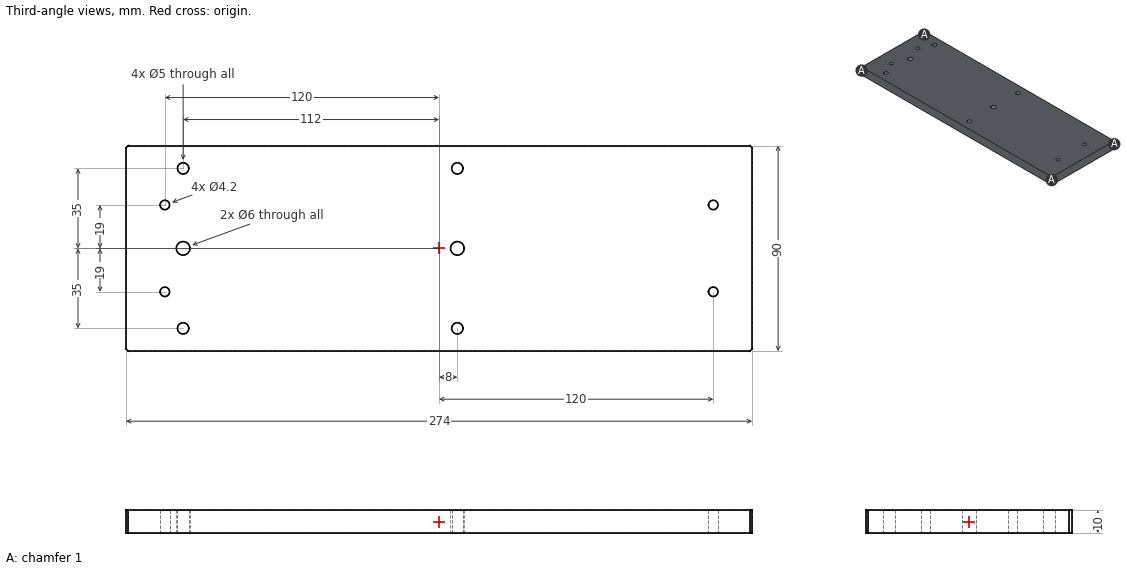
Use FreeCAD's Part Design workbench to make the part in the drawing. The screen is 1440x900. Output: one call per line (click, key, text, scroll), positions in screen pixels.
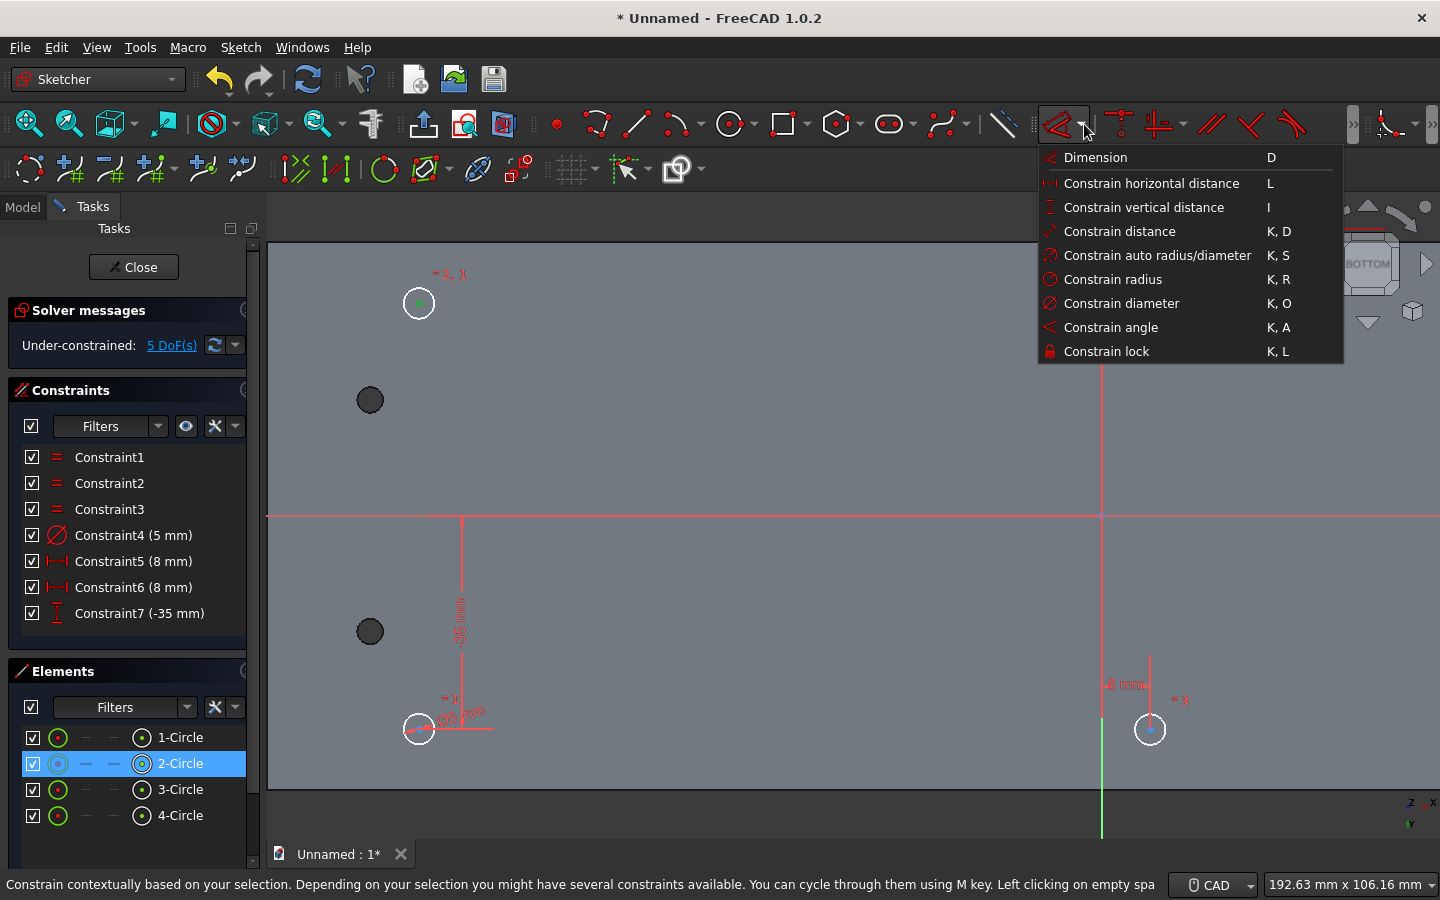
click(1191, 207)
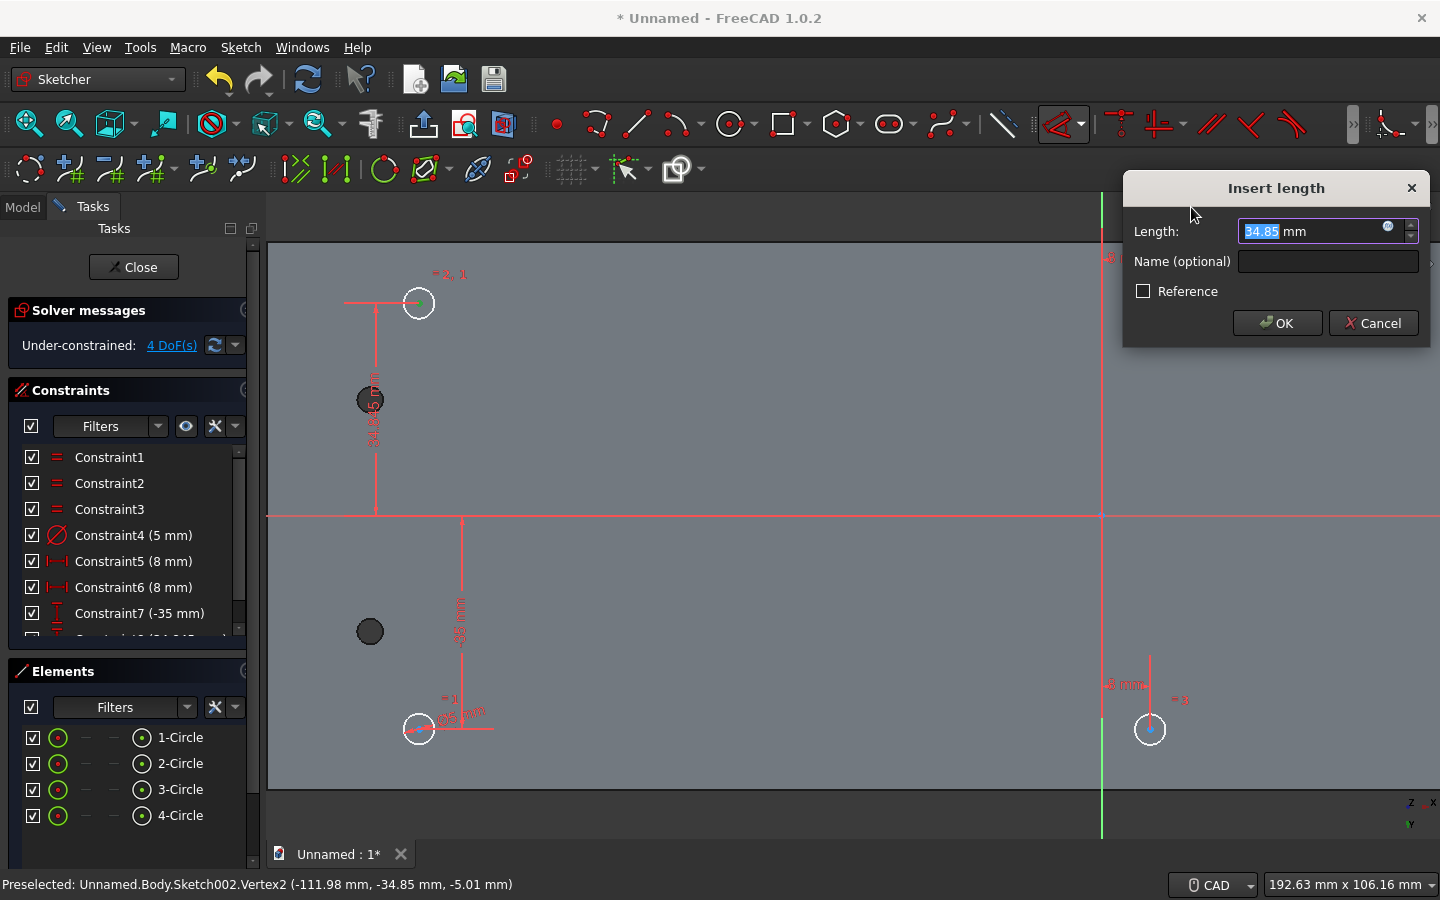
text(35)
key(Return)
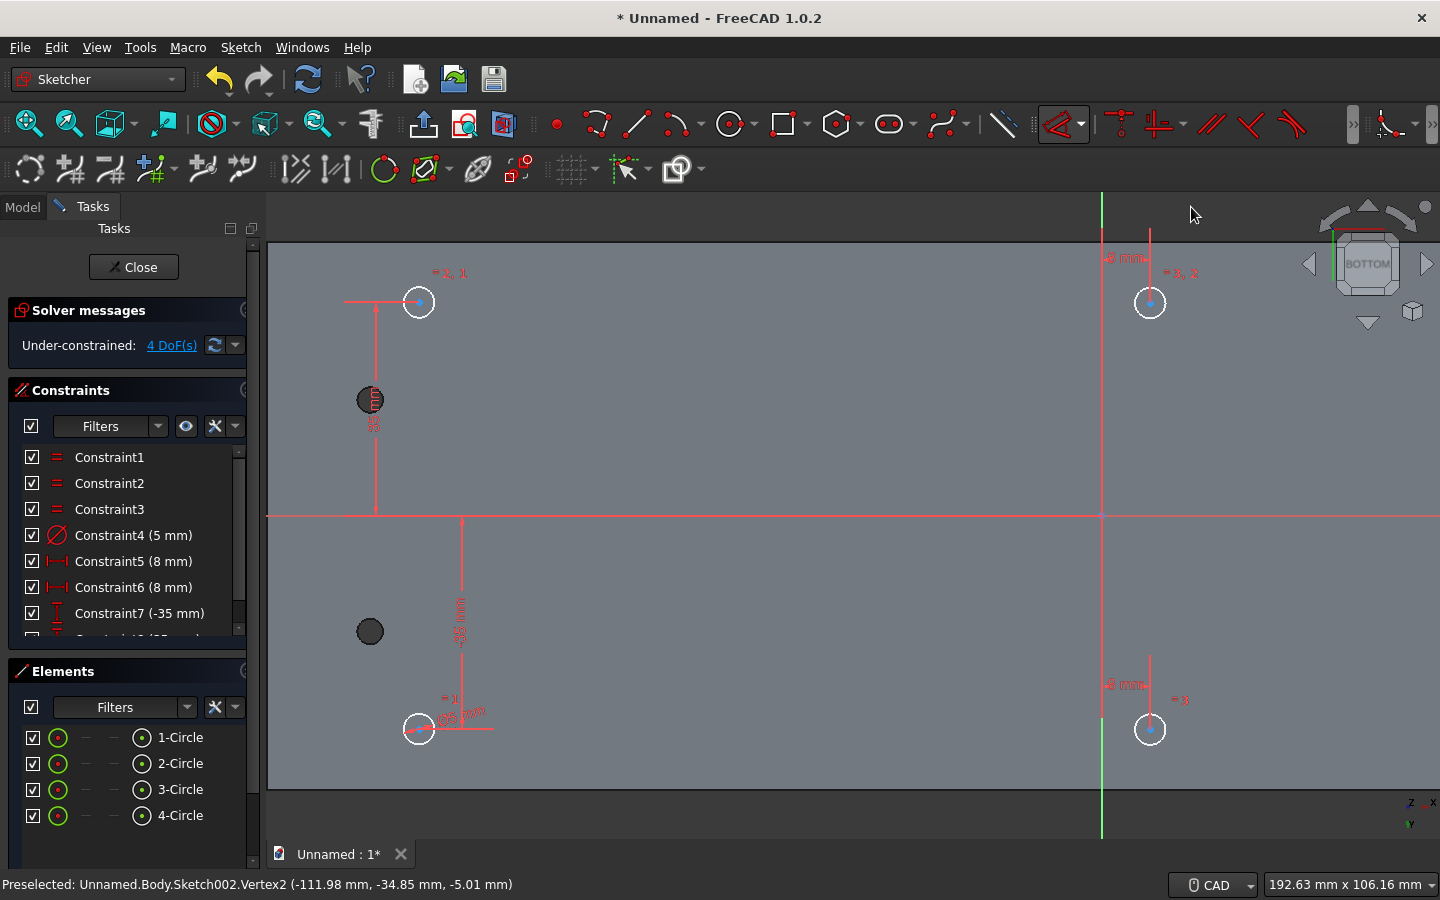
click(1150, 303)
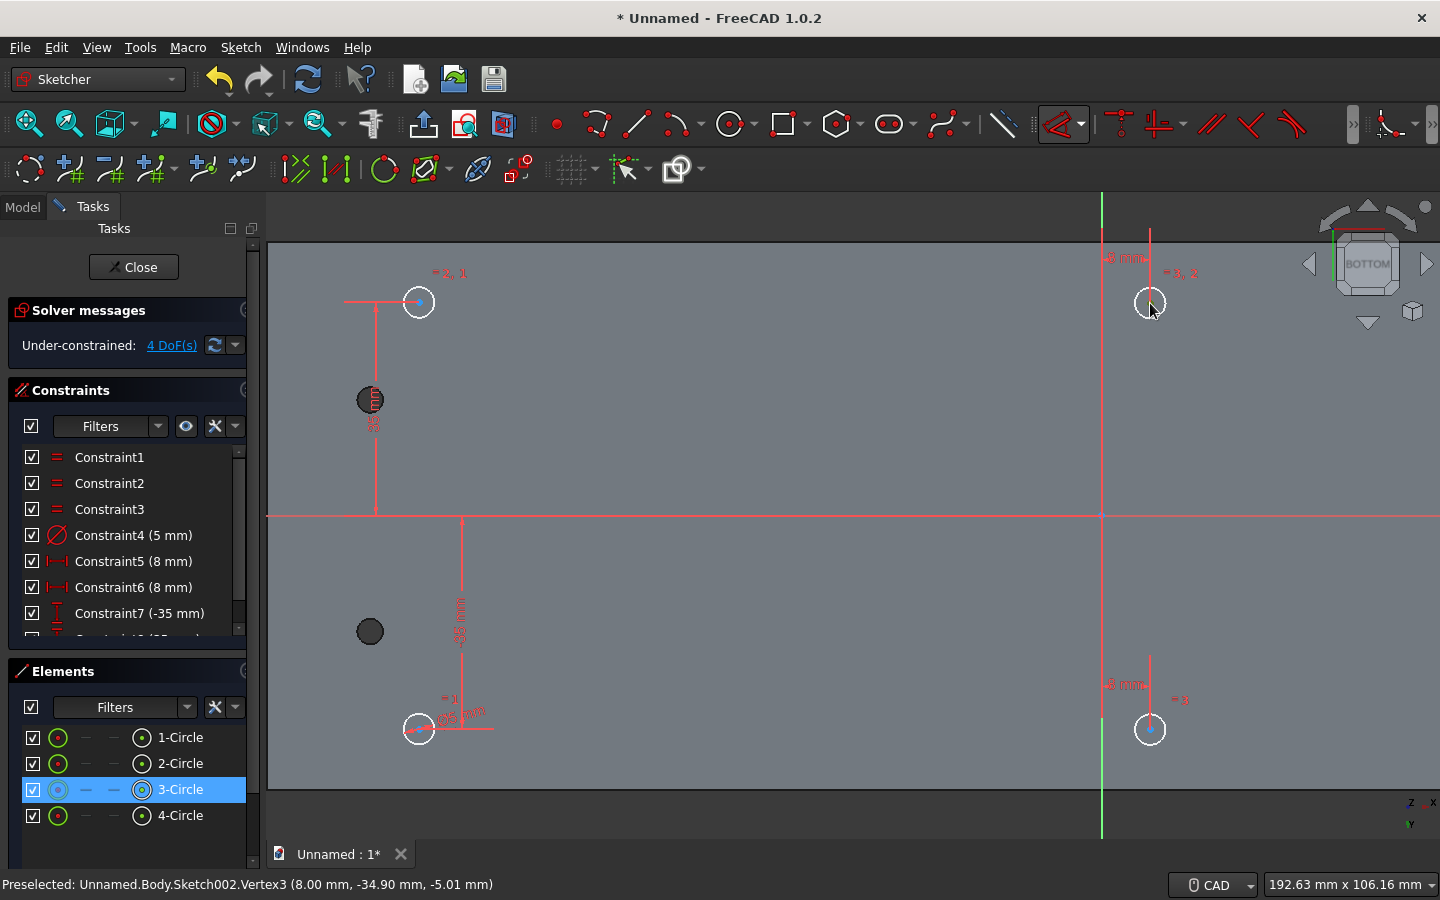
key(i)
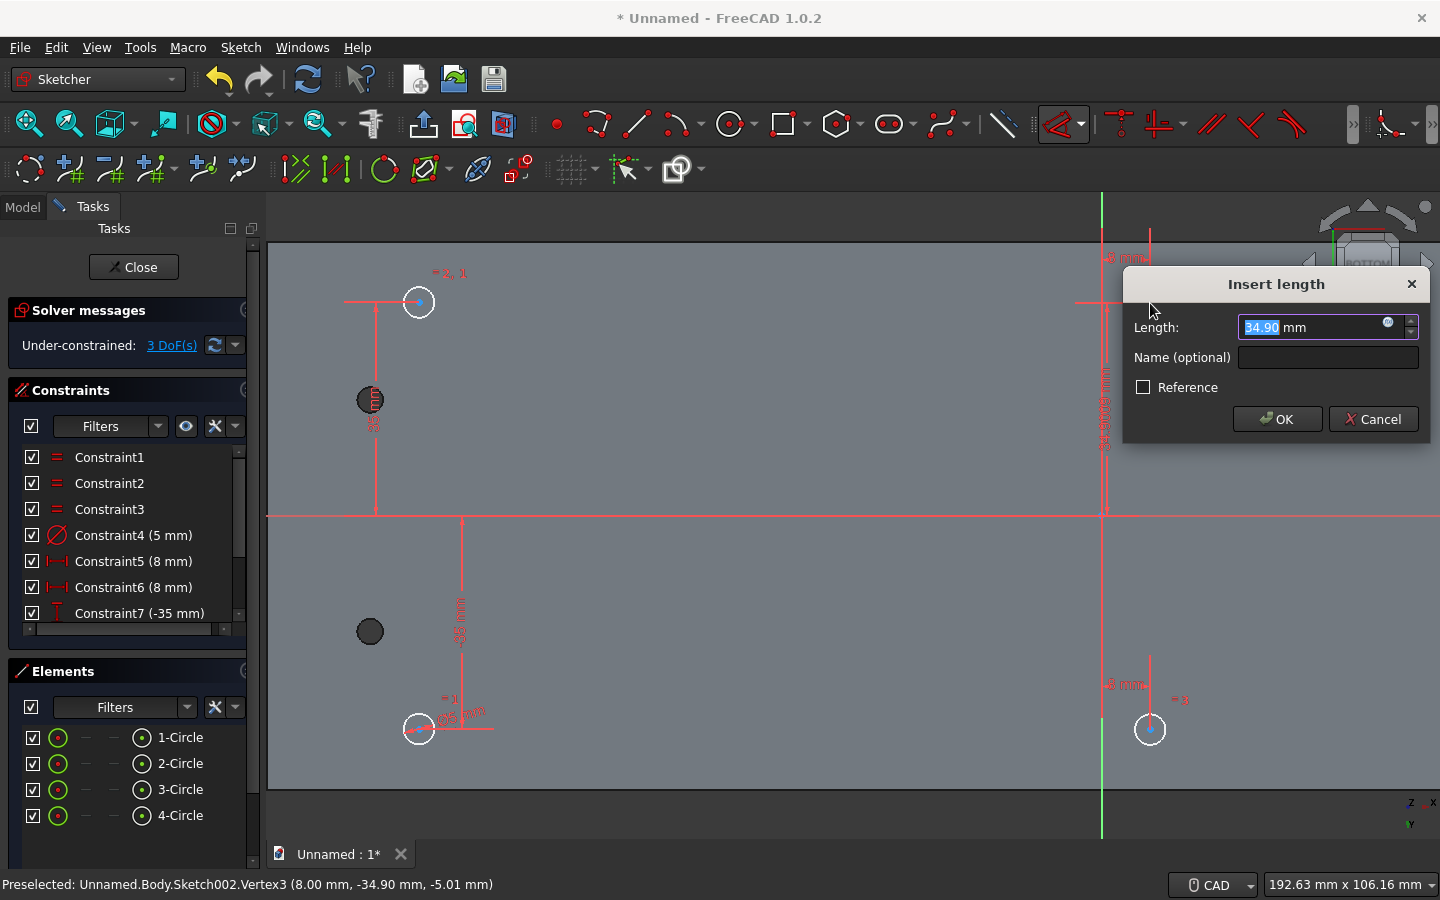
text(35)
key(Return)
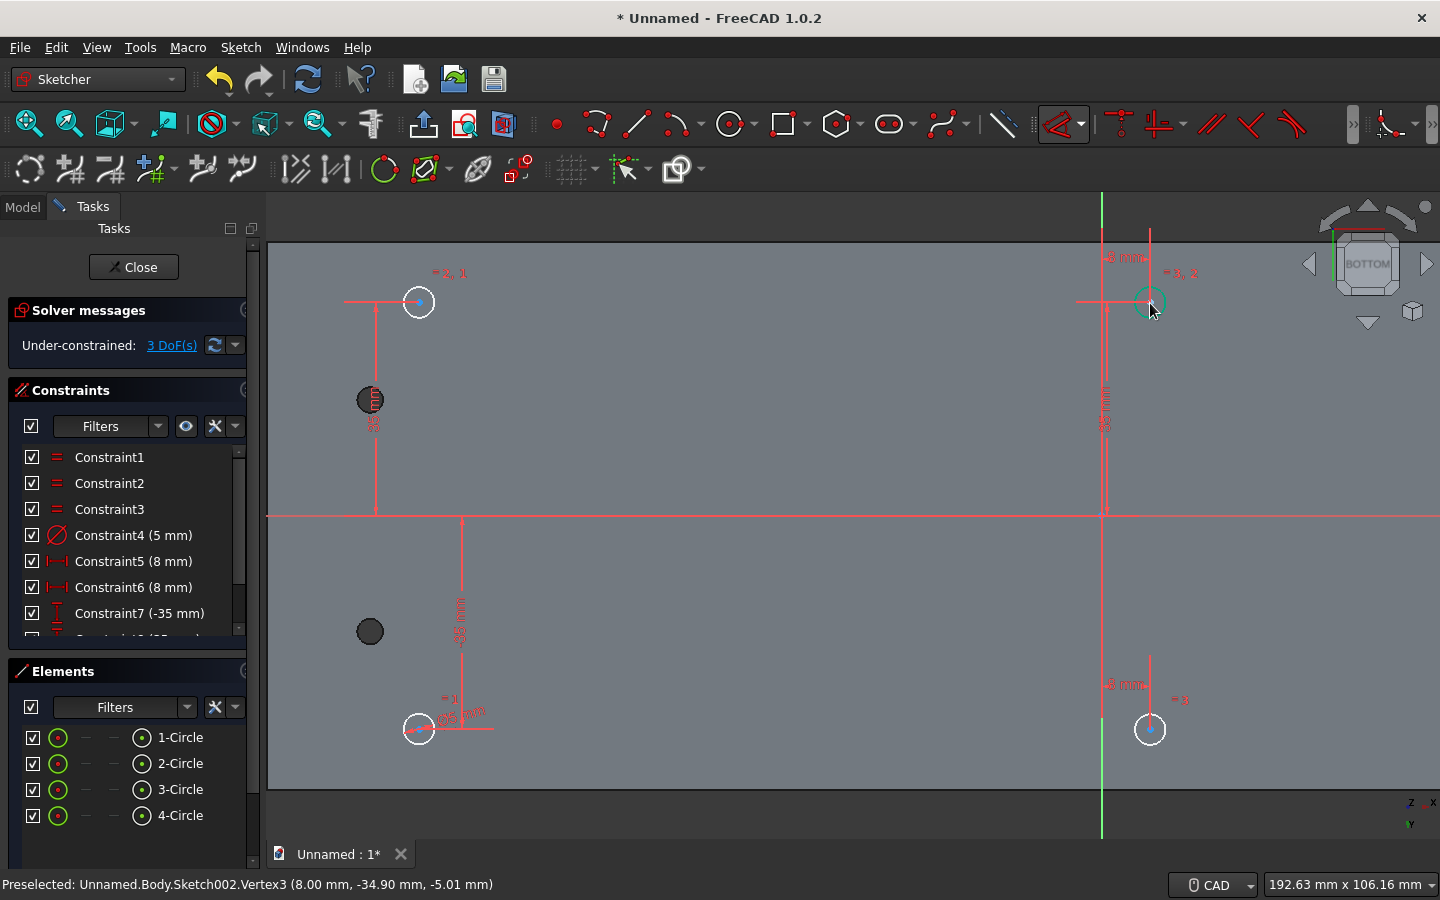
click(1150, 730)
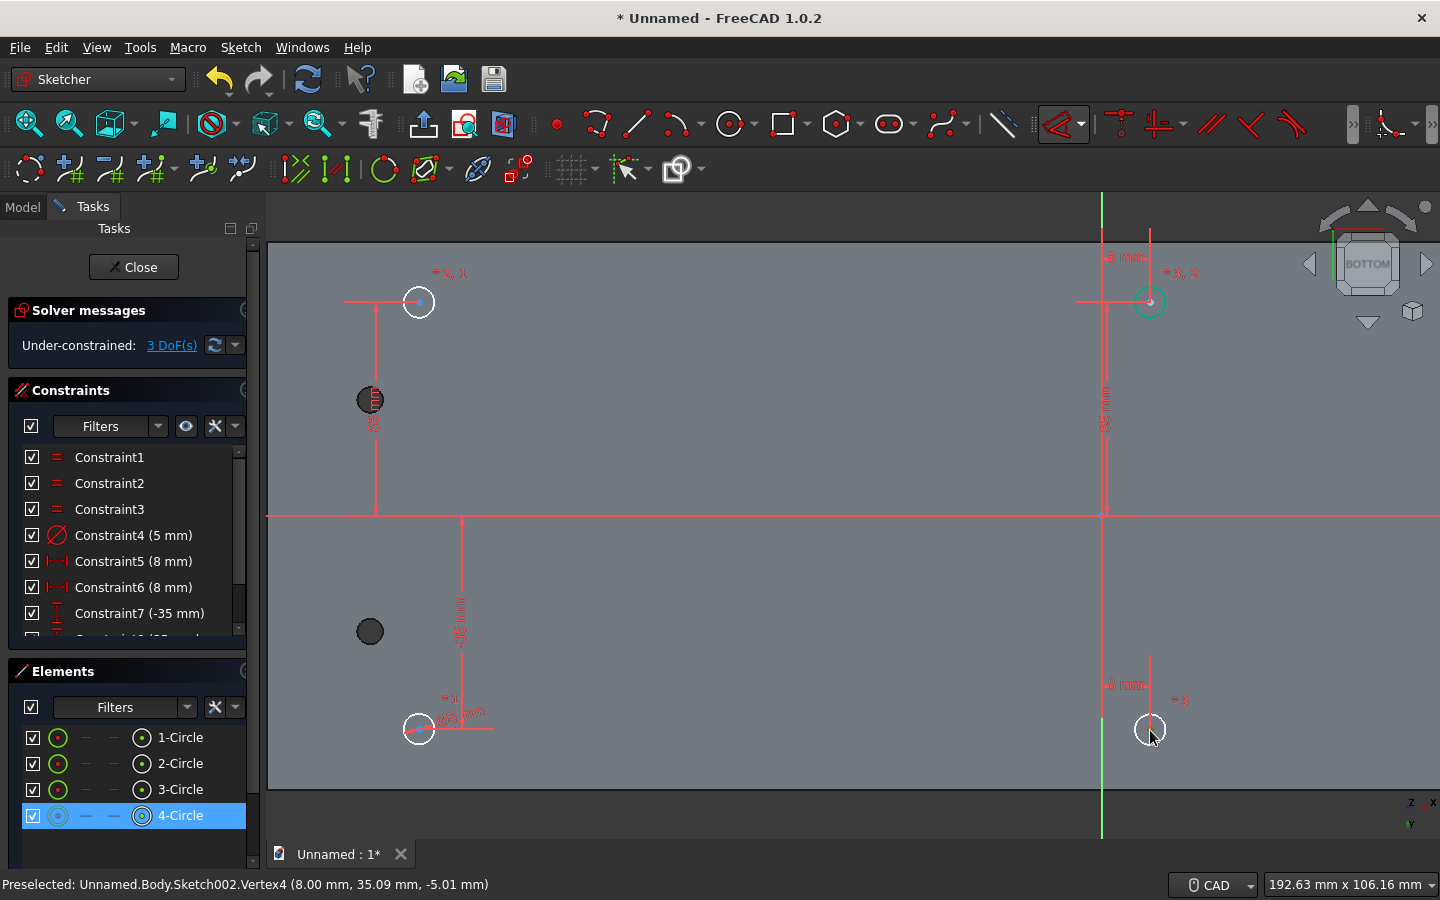
key(i)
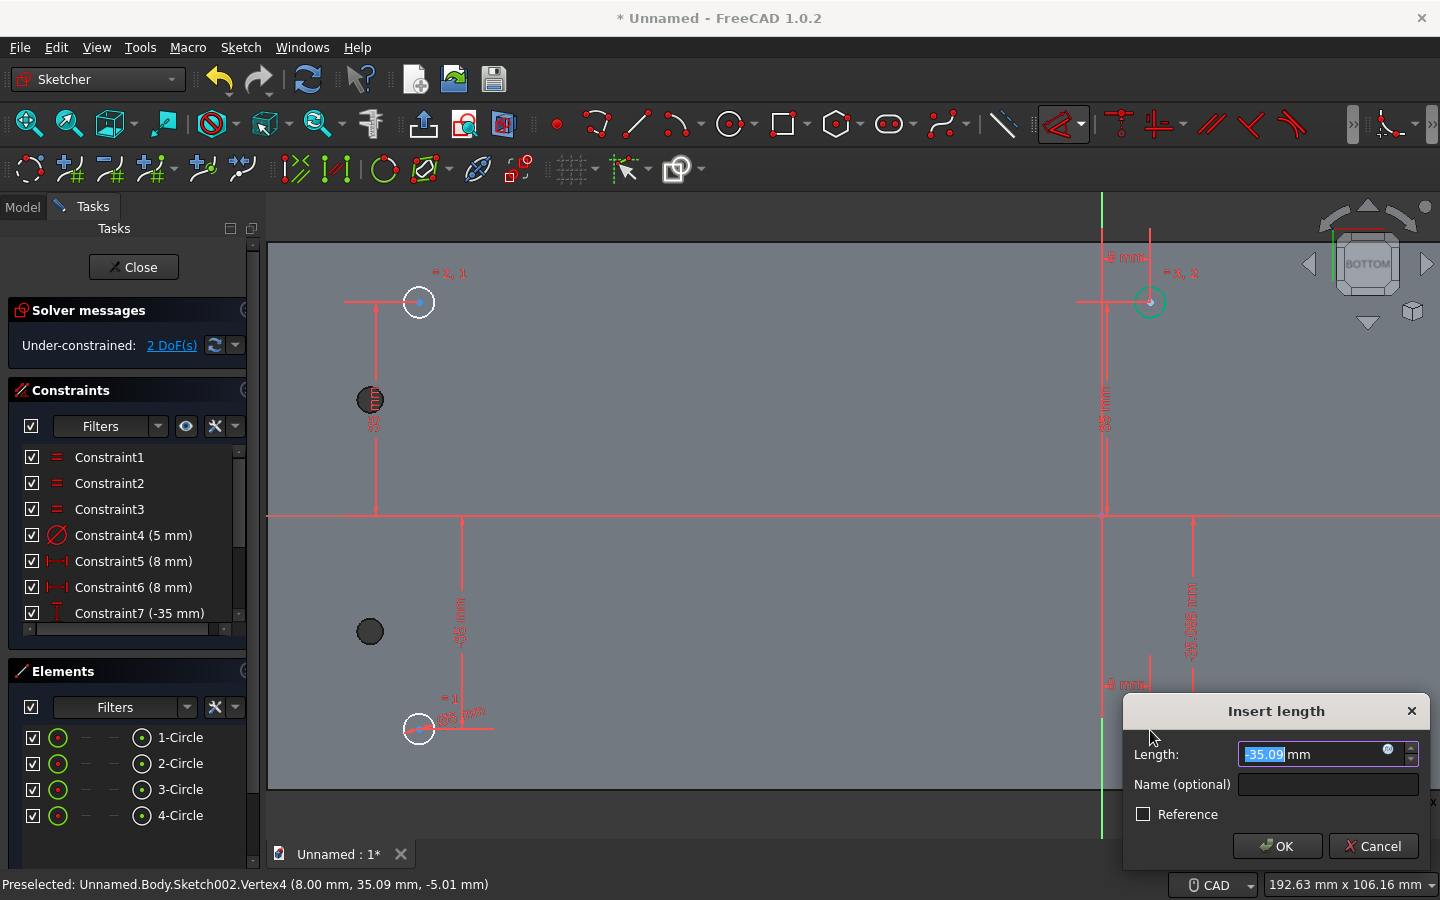
text(-35)
key(Return)